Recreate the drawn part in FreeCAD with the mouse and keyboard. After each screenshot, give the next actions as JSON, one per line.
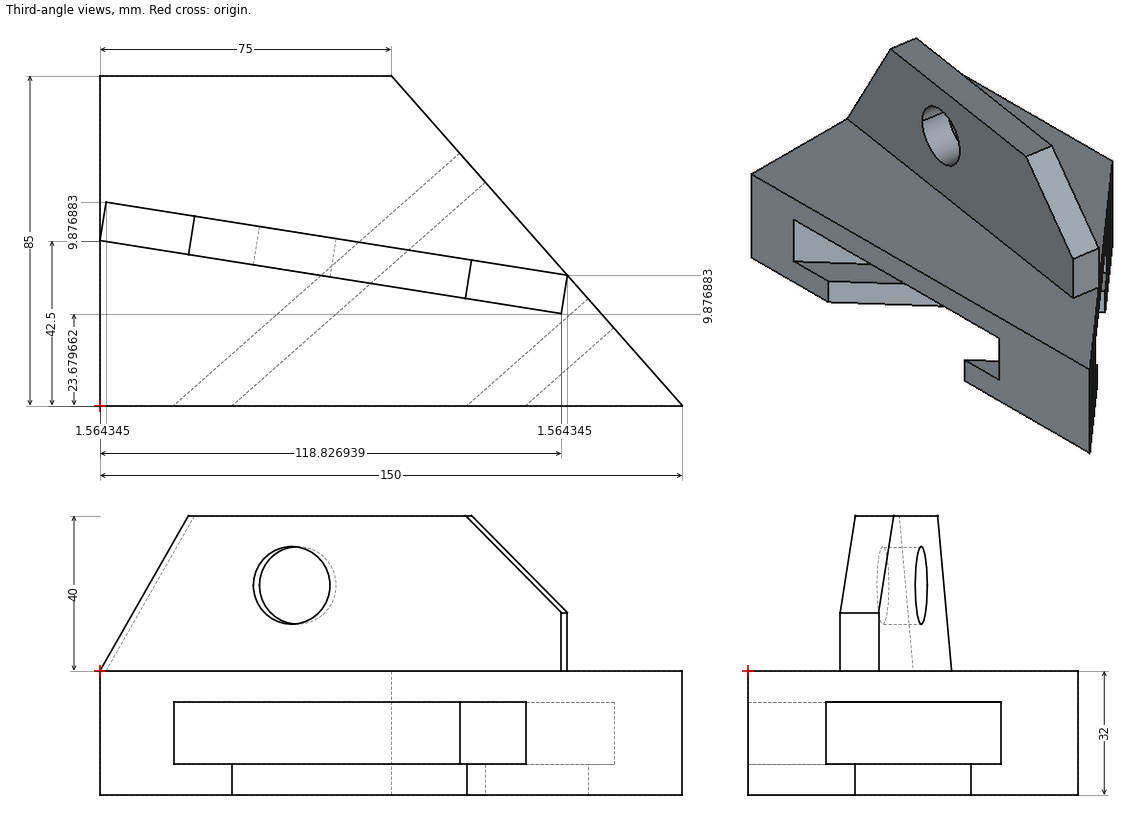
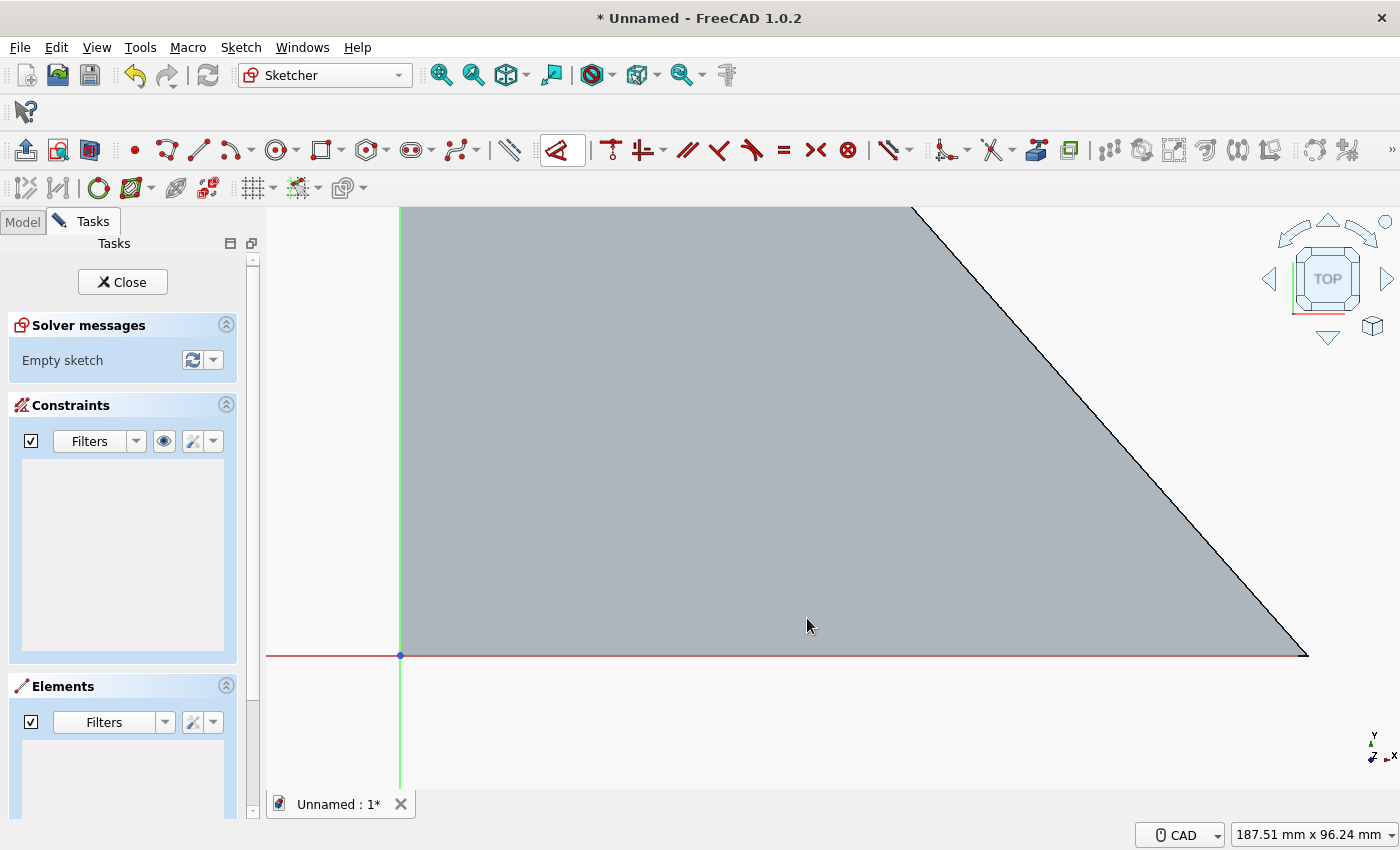
{"action": "key", "text": "g m"}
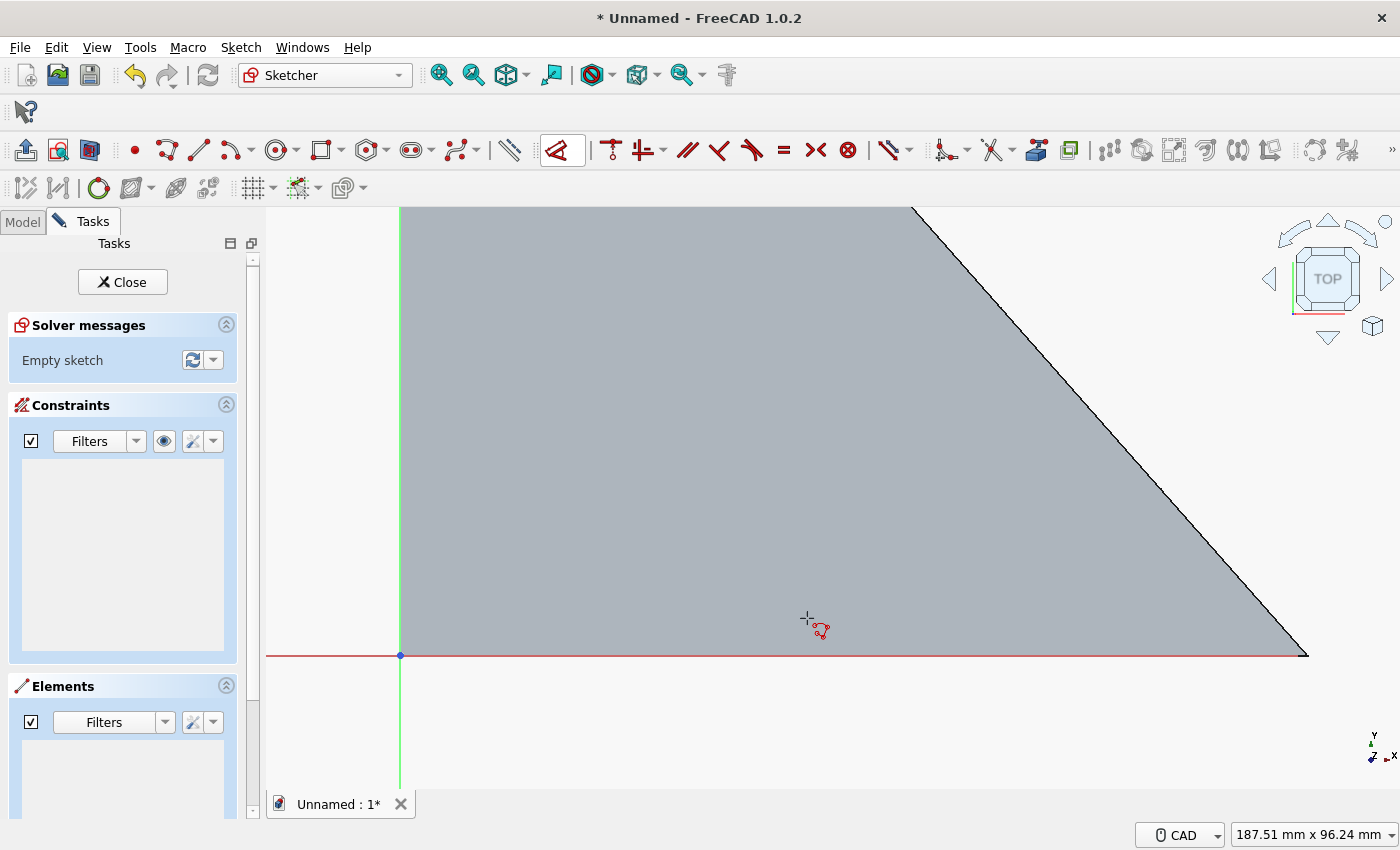
{"action": "left_click", "coordinate": [400, 399]}
{"action": "left_click", "coordinate": [1119, 513]}
{"action": "left_click", "coordinate": [1128, 453]}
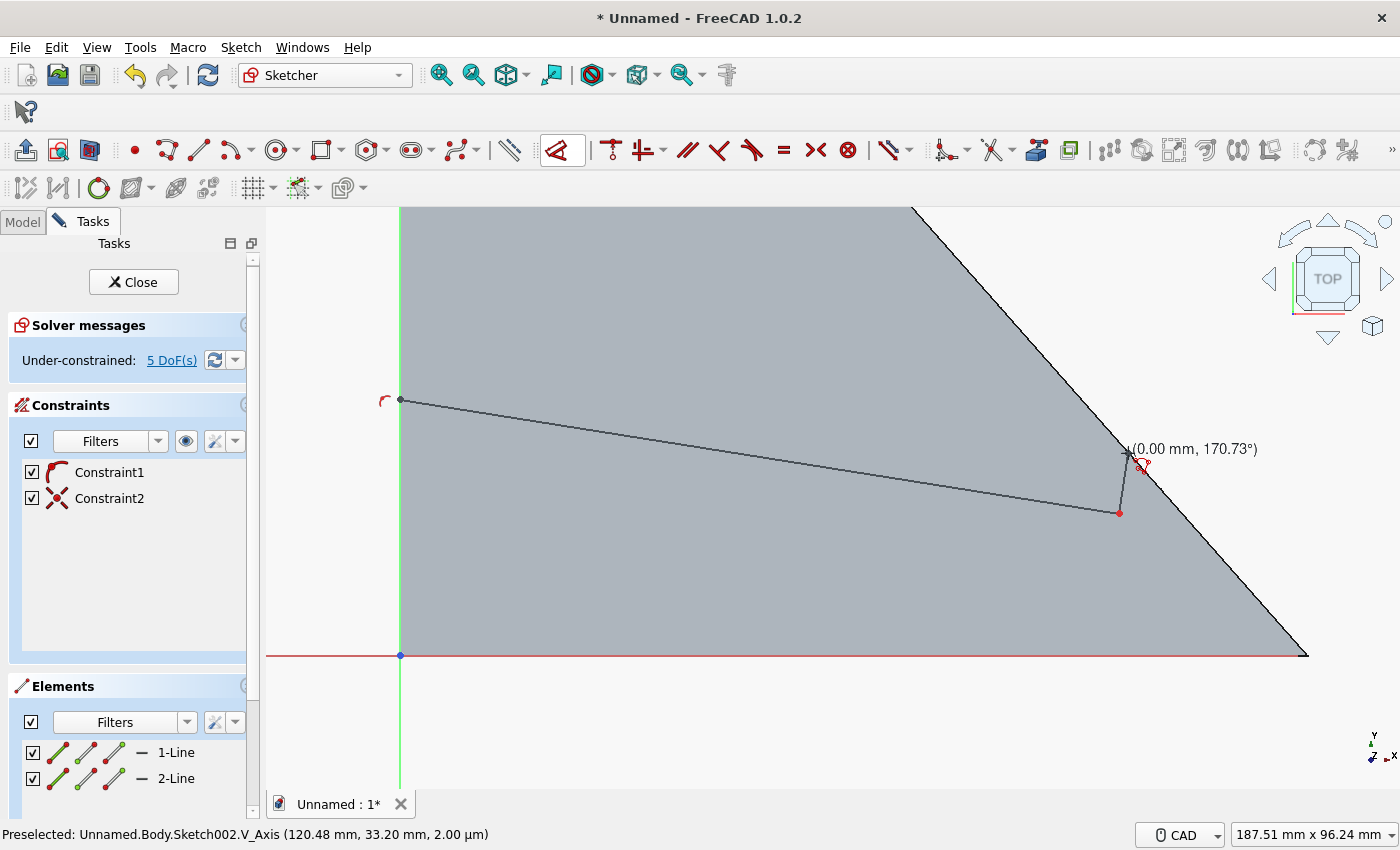
{"action": "scroll", "coordinate": [410, 339], "scroll_direction": "up", "scroll_amount": 3}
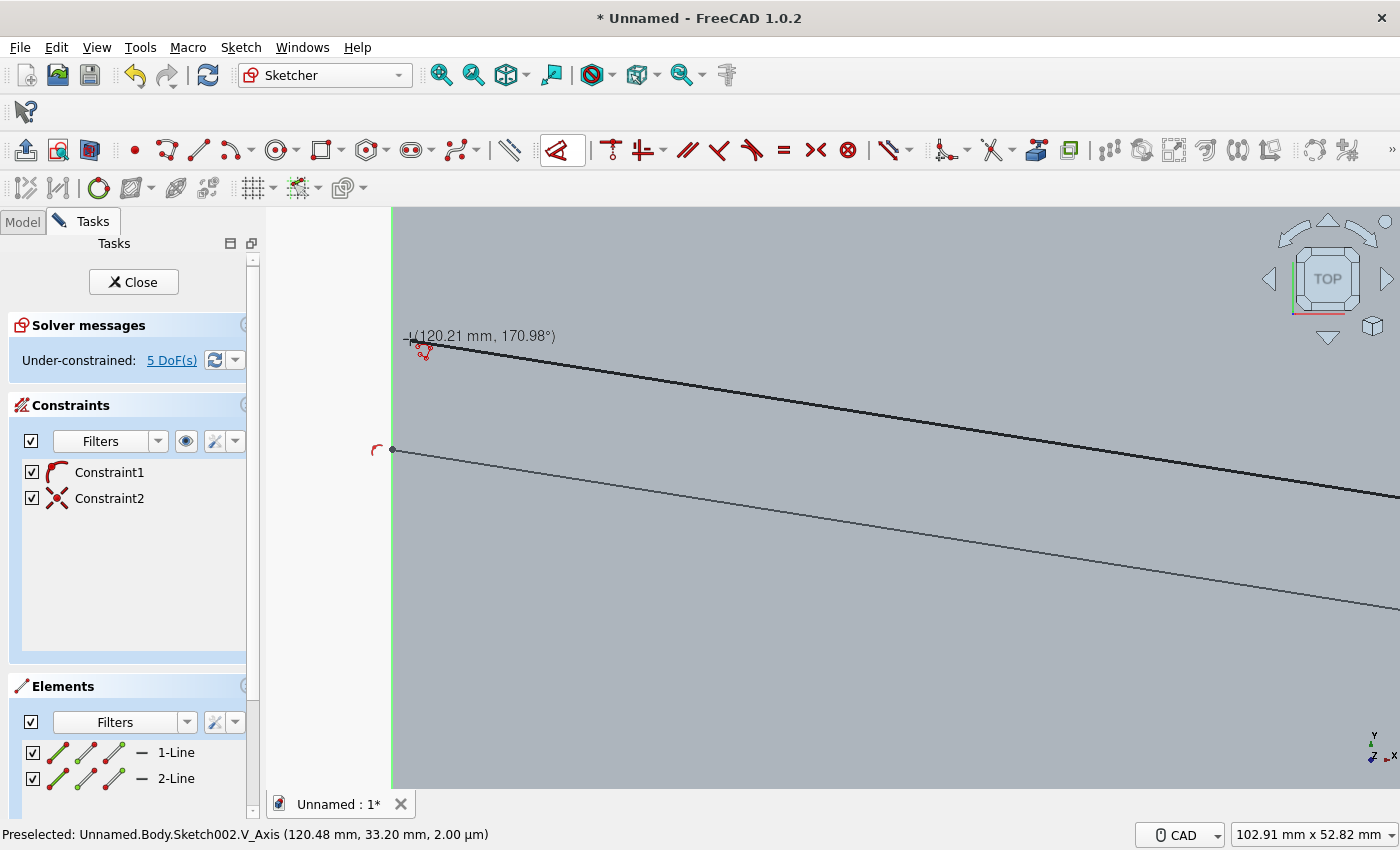
{"action": "left_click", "coordinate": [410, 339]}
{"action": "left_click", "coordinate": [392, 450]}
{"action": "key", "text": "Escape"}
{"action": "key", "text": "Escape"}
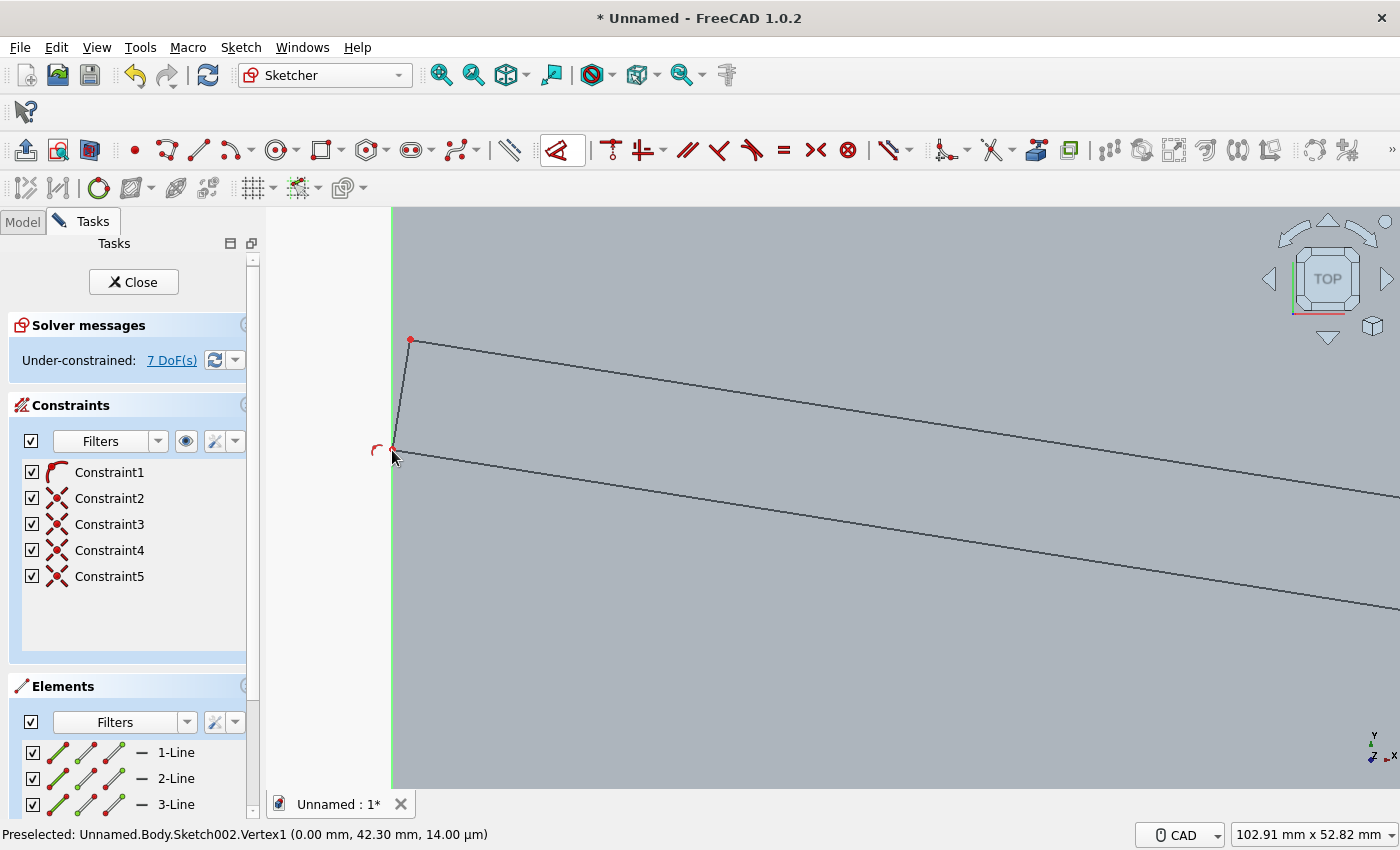
{"action": "left_click", "coordinate": [392, 450]}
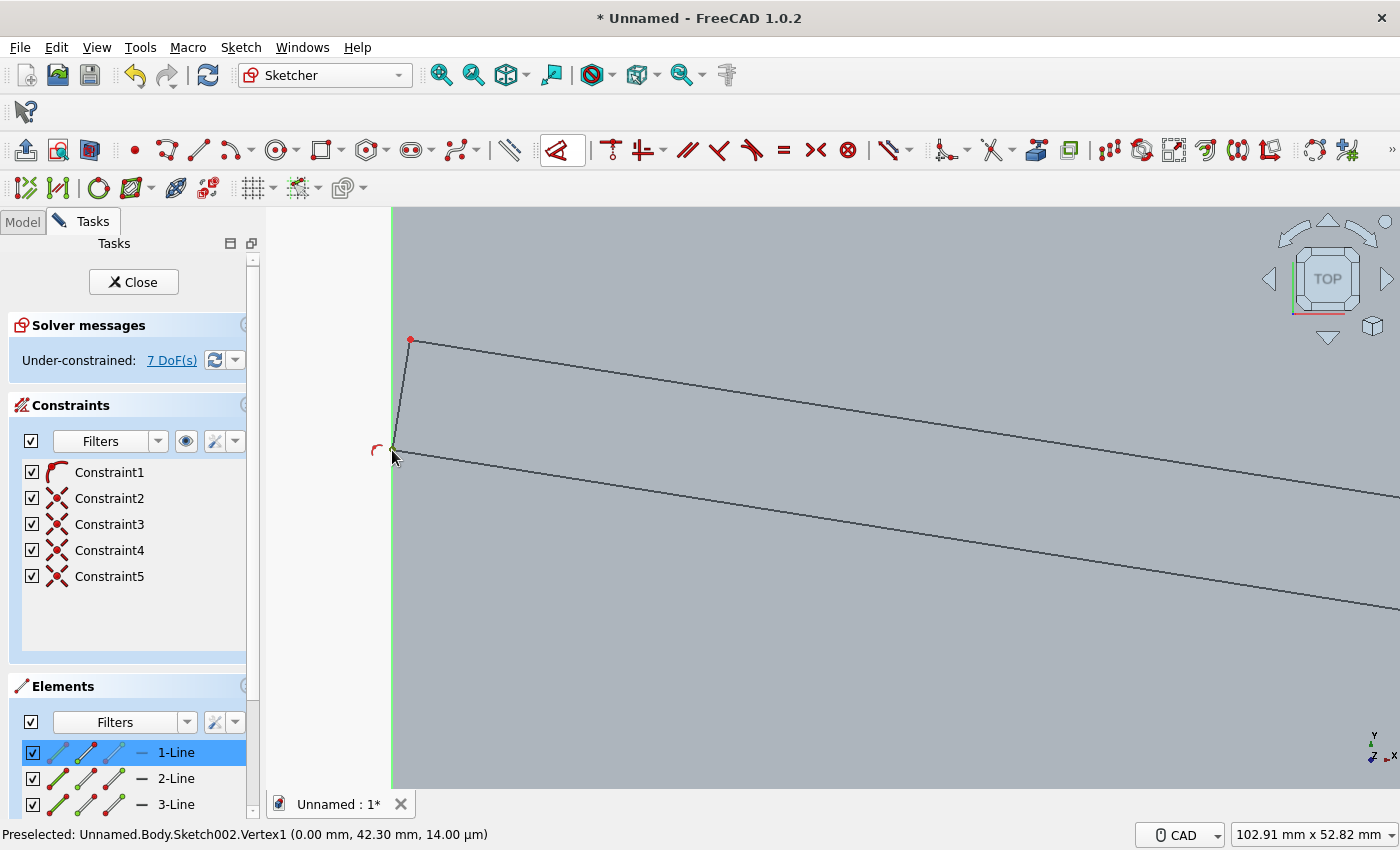
{"action": "key", "text": "i"}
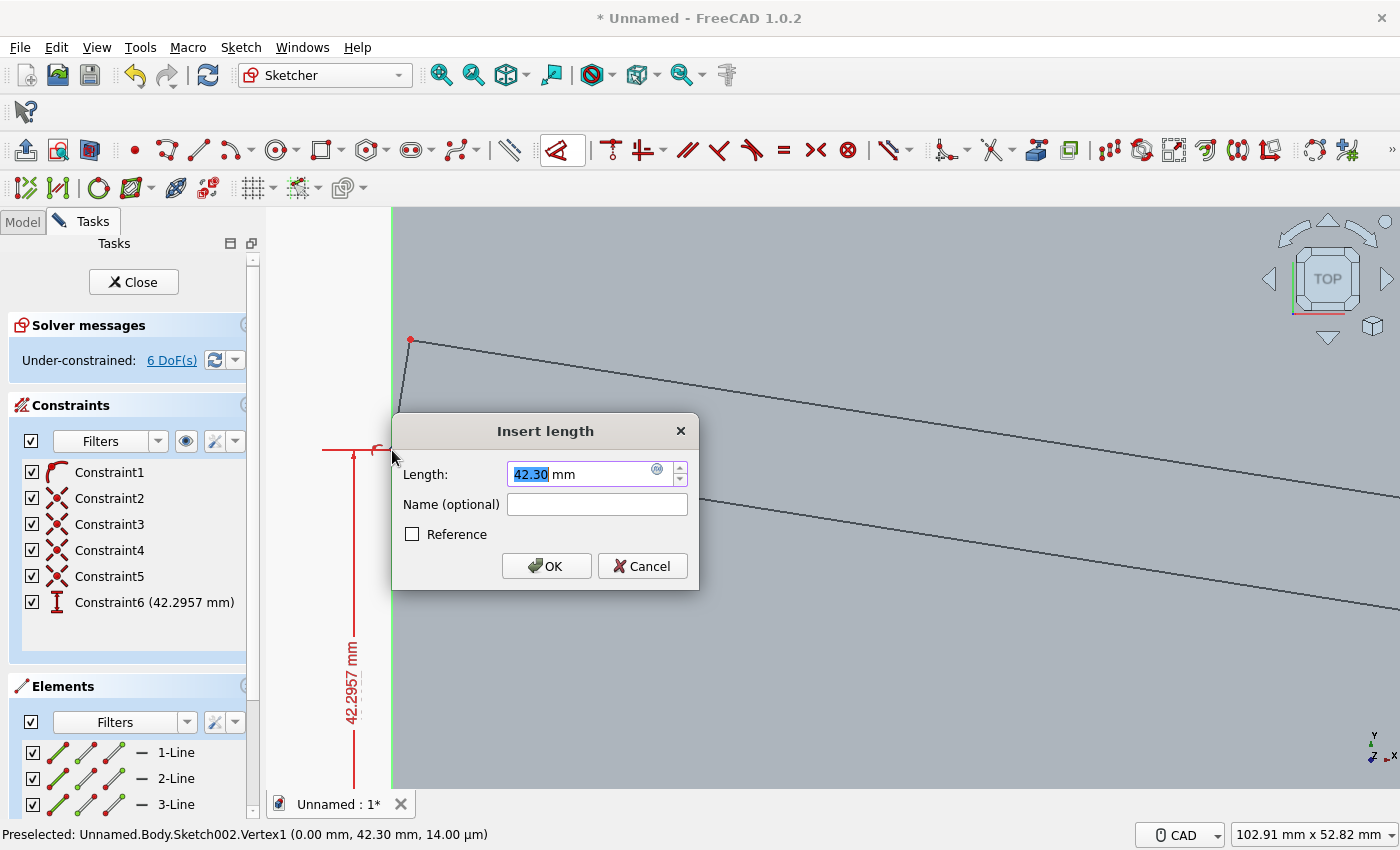
{"action": "type", "text": "42.5"}
{"action": "key", "text": "Return"}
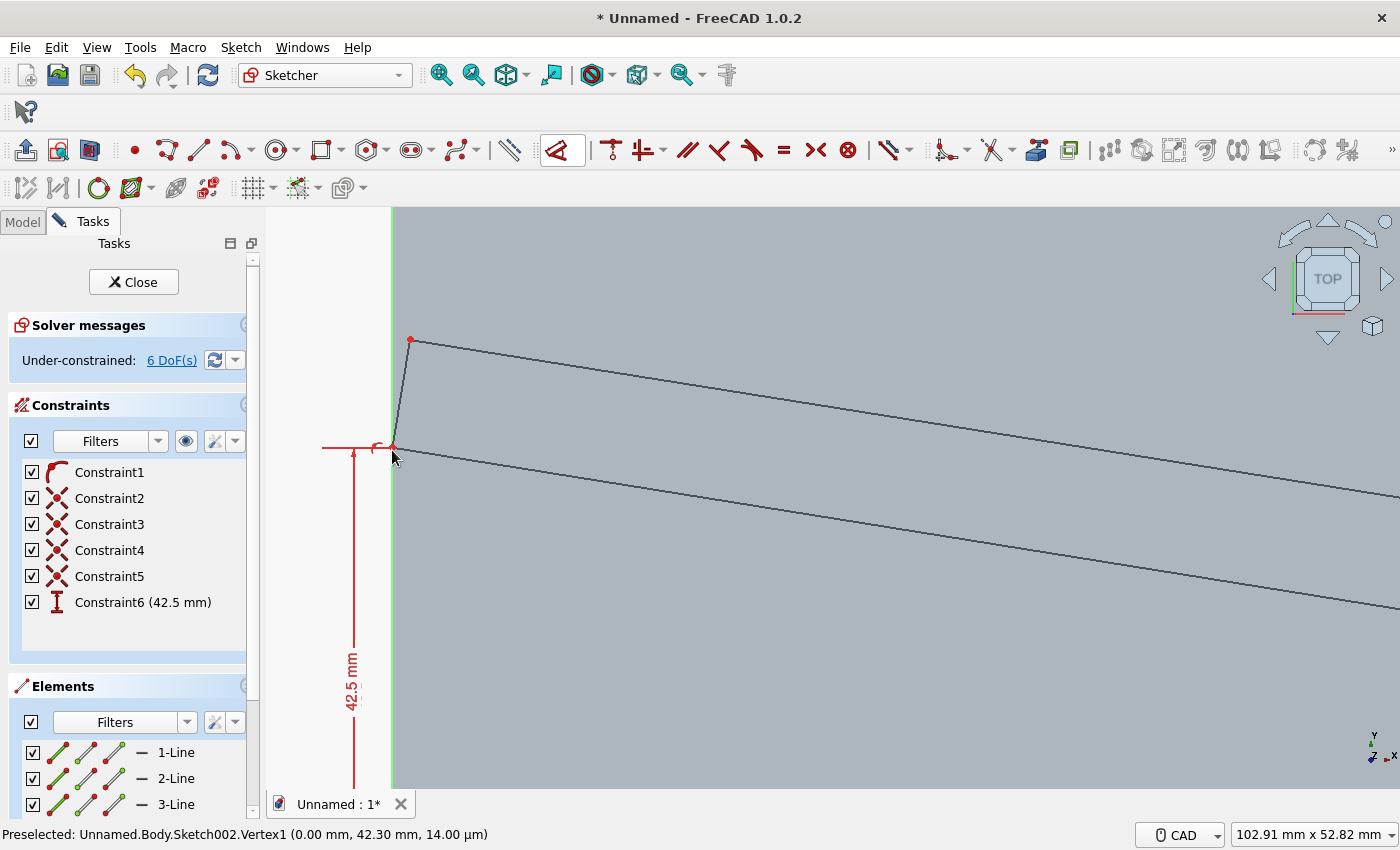
{"action": "scroll", "coordinate": [410, 340], "scroll_direction": "up", "scroll_amount": 5}